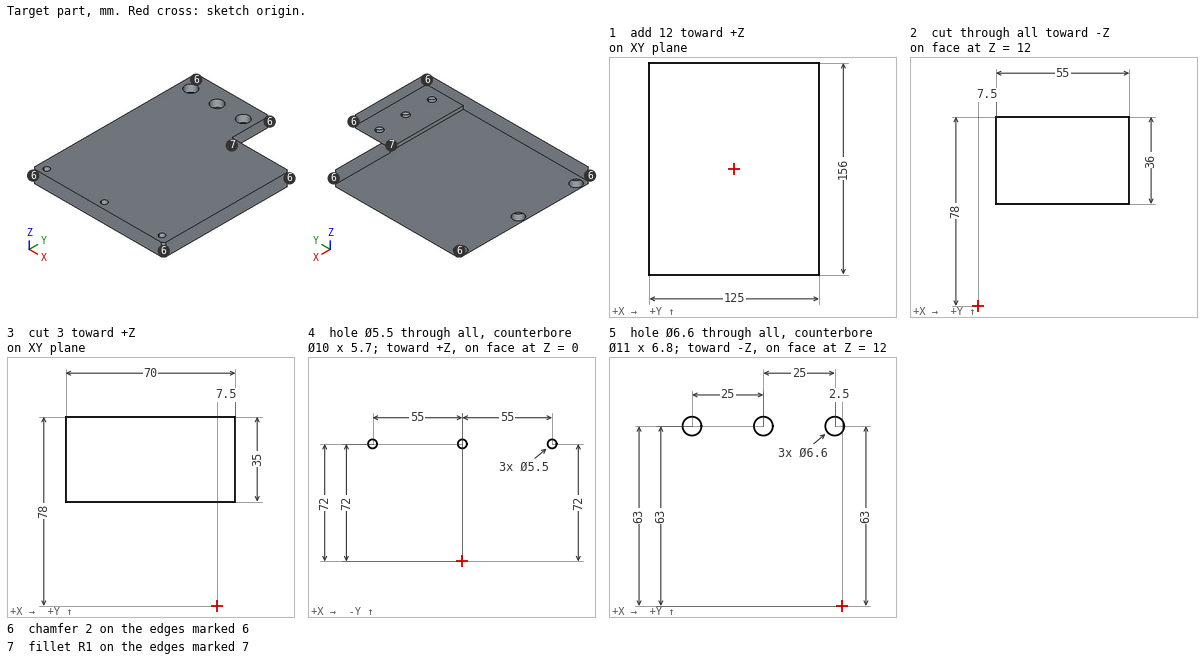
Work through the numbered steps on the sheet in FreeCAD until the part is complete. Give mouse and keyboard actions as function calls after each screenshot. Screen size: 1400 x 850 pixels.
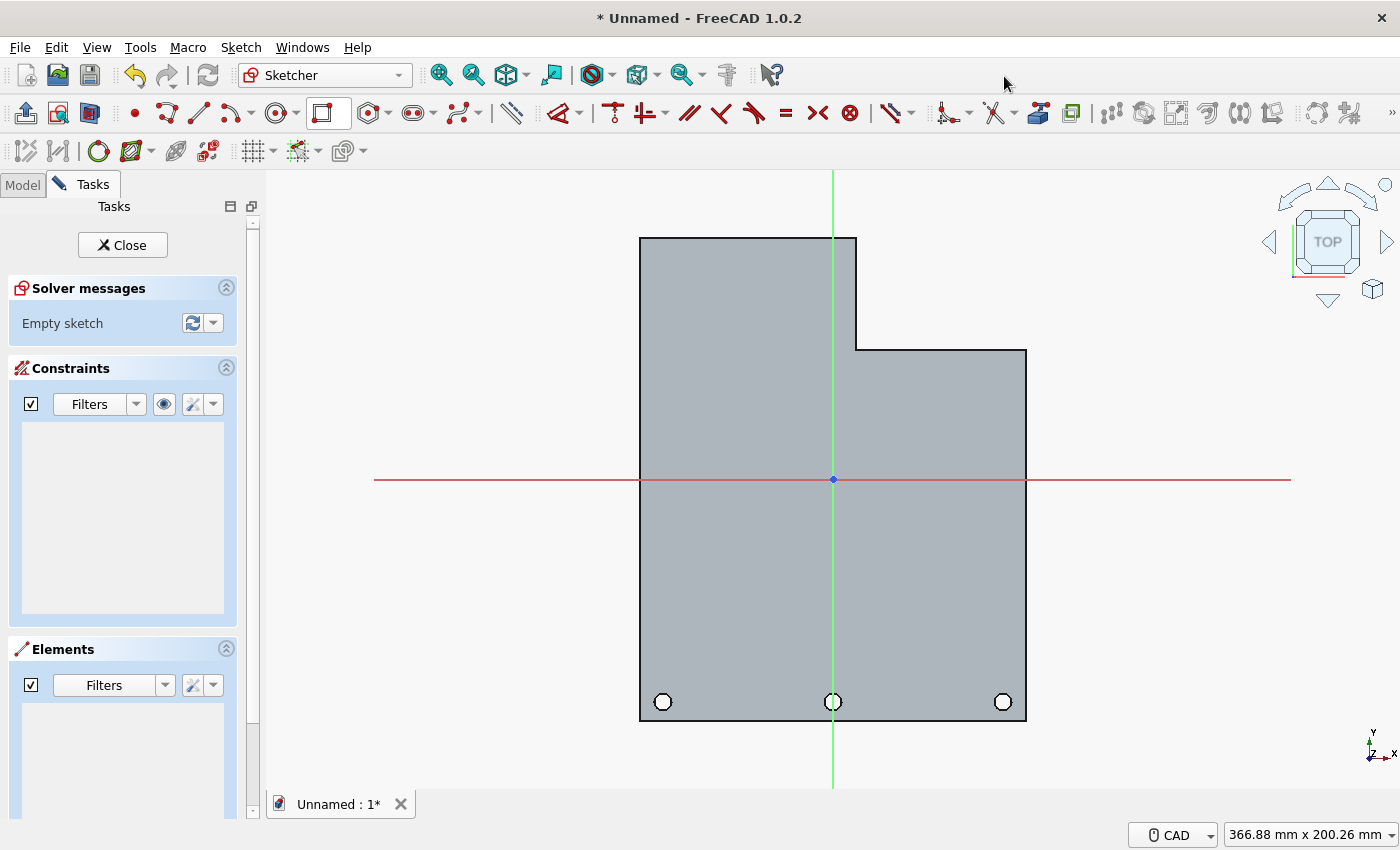
scroll(728, 252, up, 3)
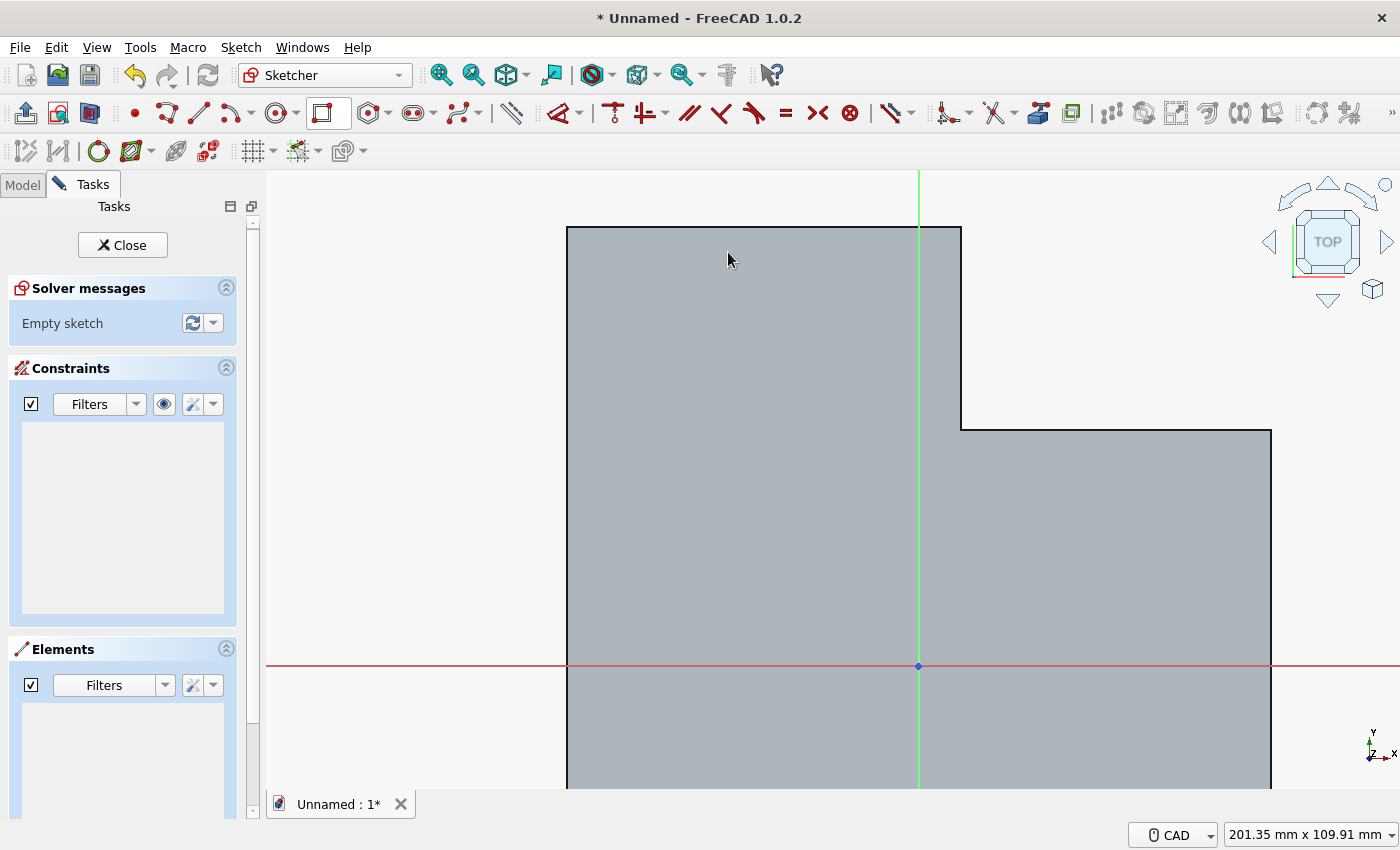
click(276, 114)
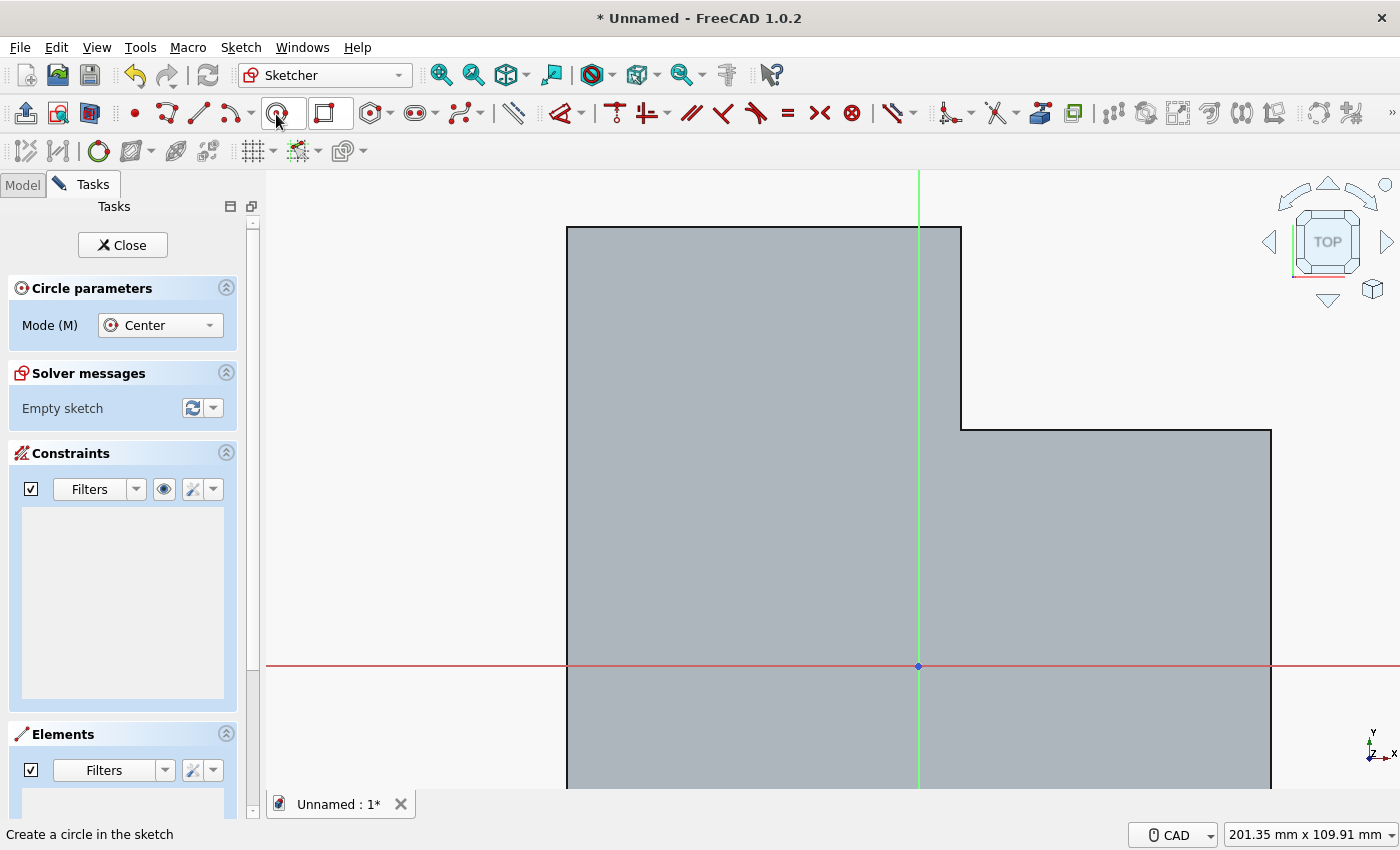
click(905, 312)
move(892, 298)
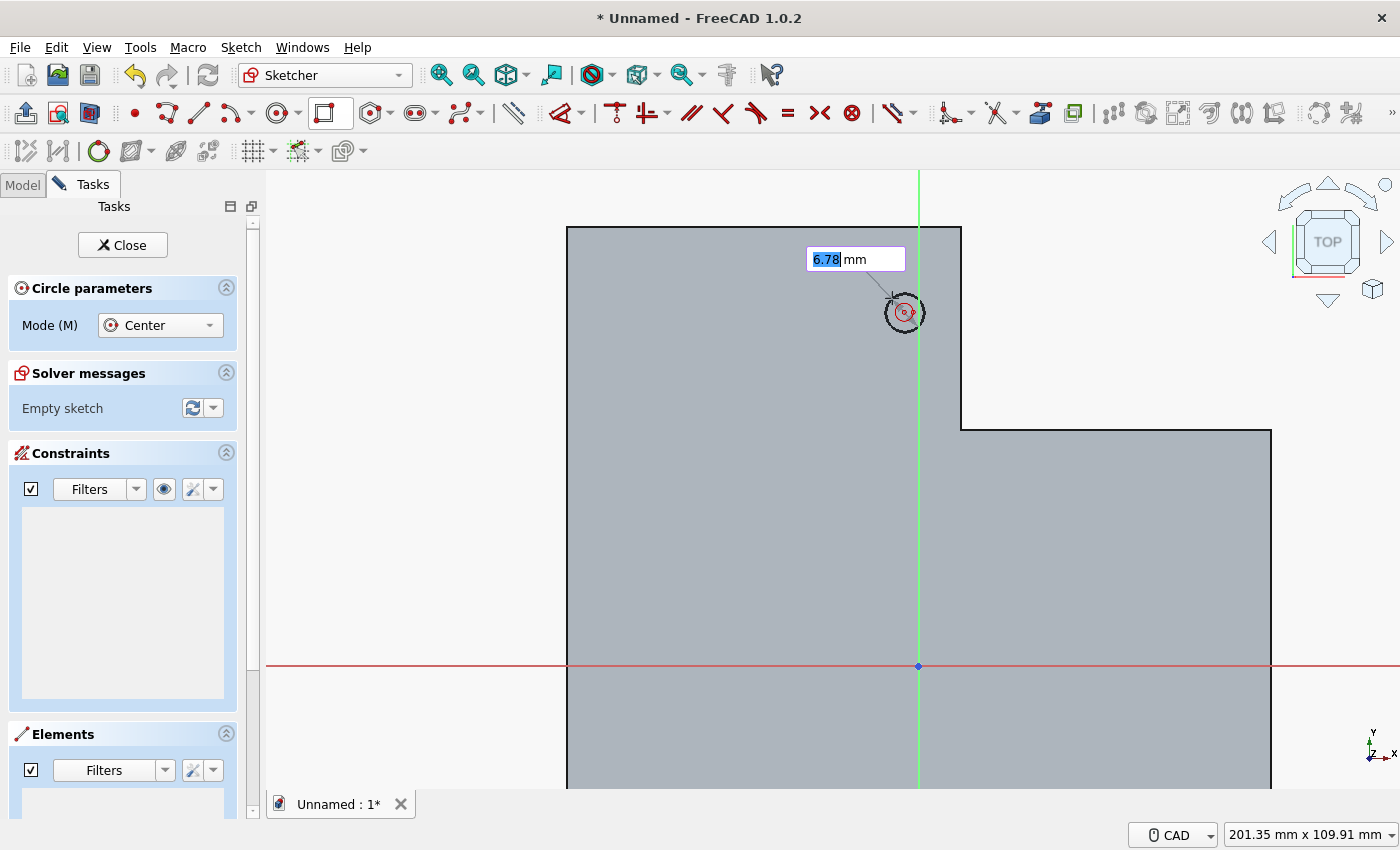
text(6.6)
key(Return)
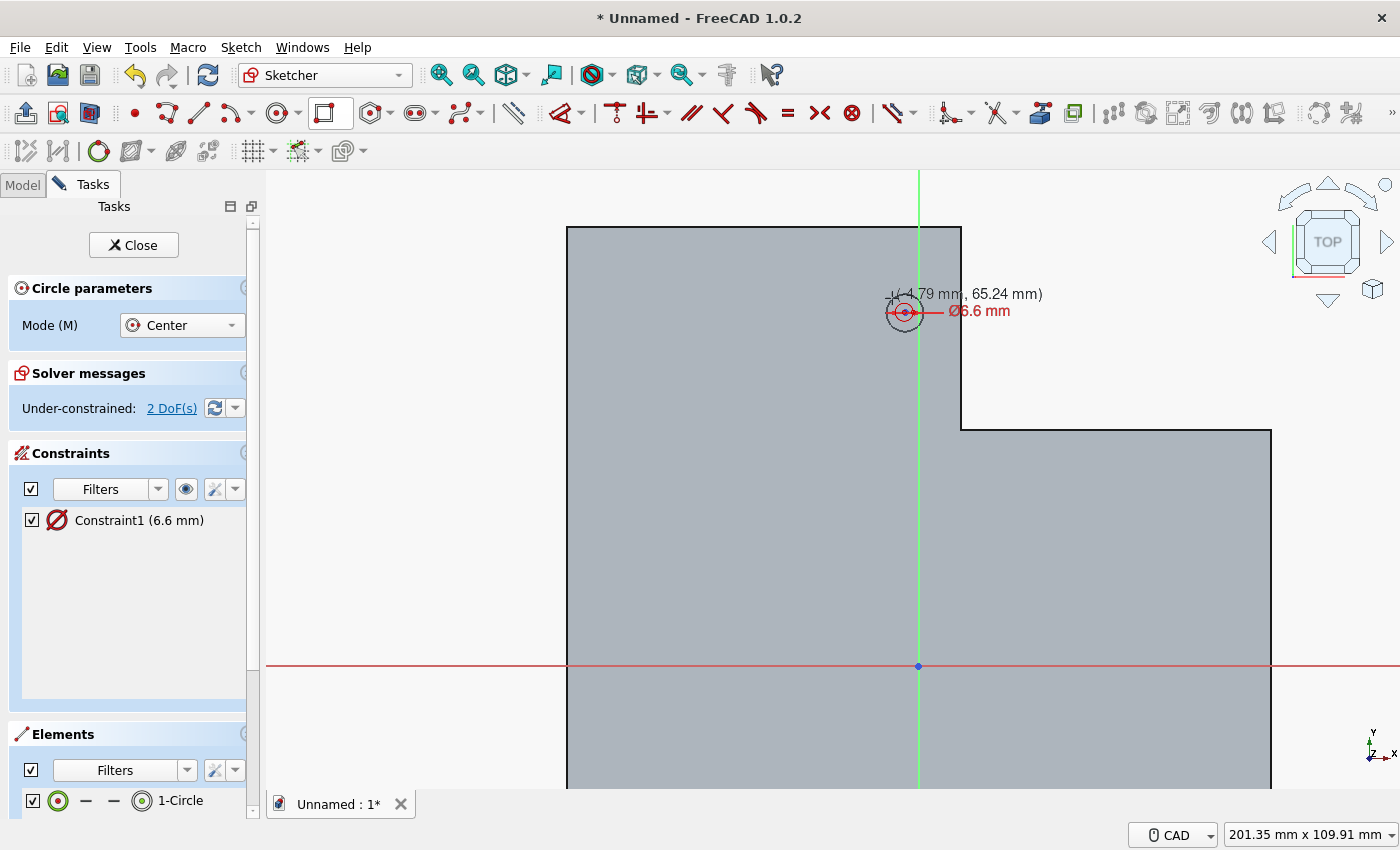
click(764, 312)
move(777, 298)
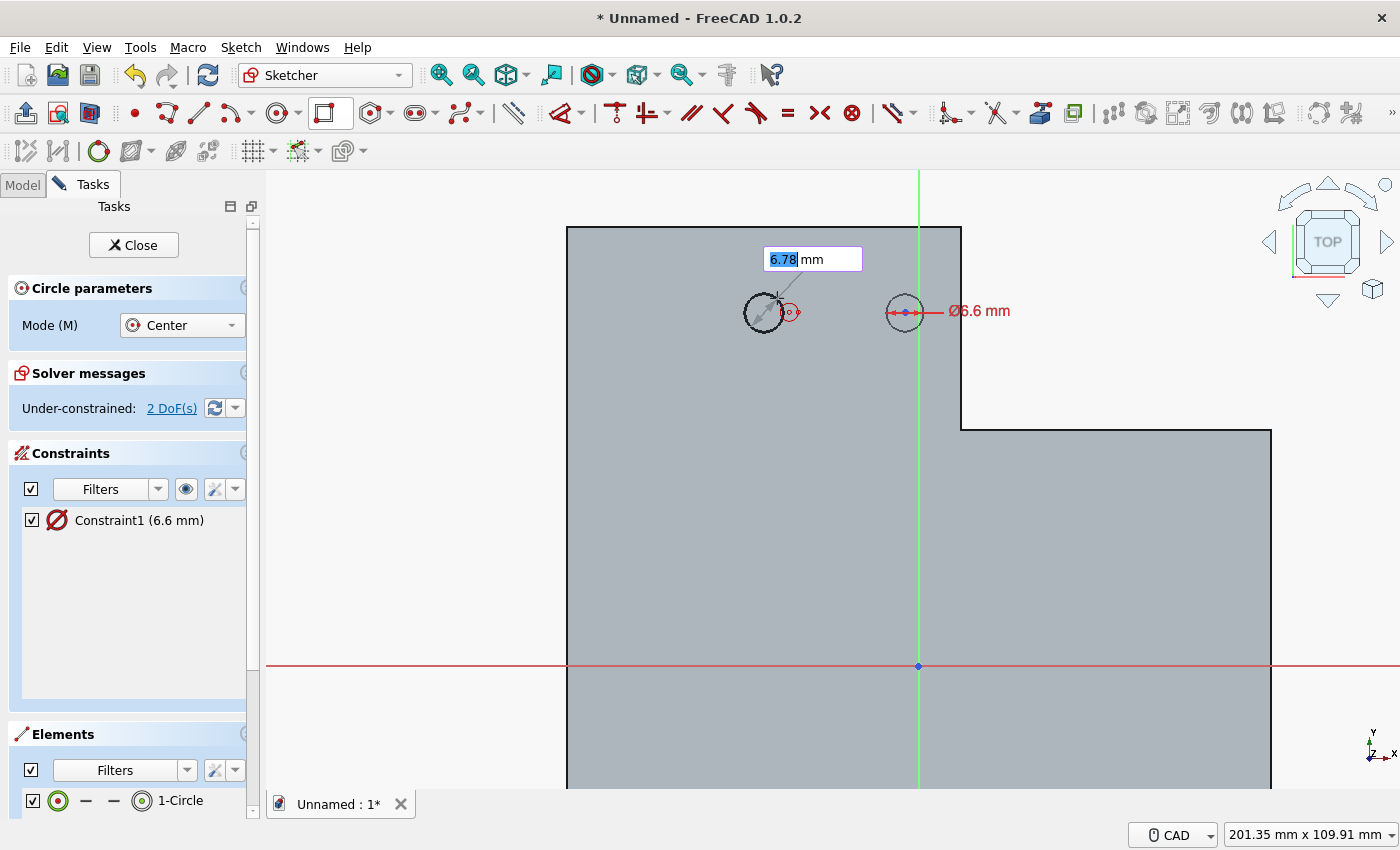
text(6.6)
key(Return)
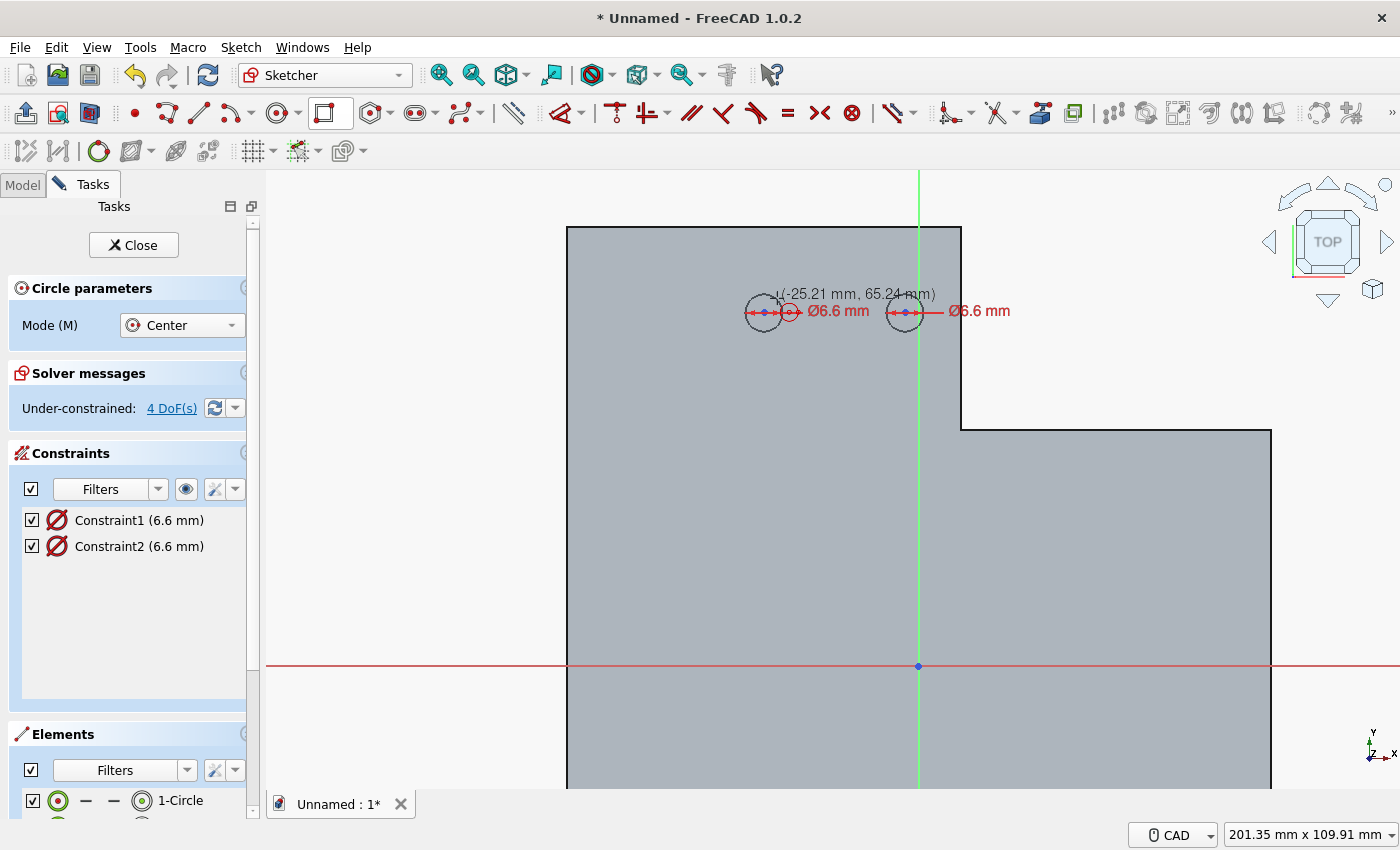
click(623, 312)
move(636, 298)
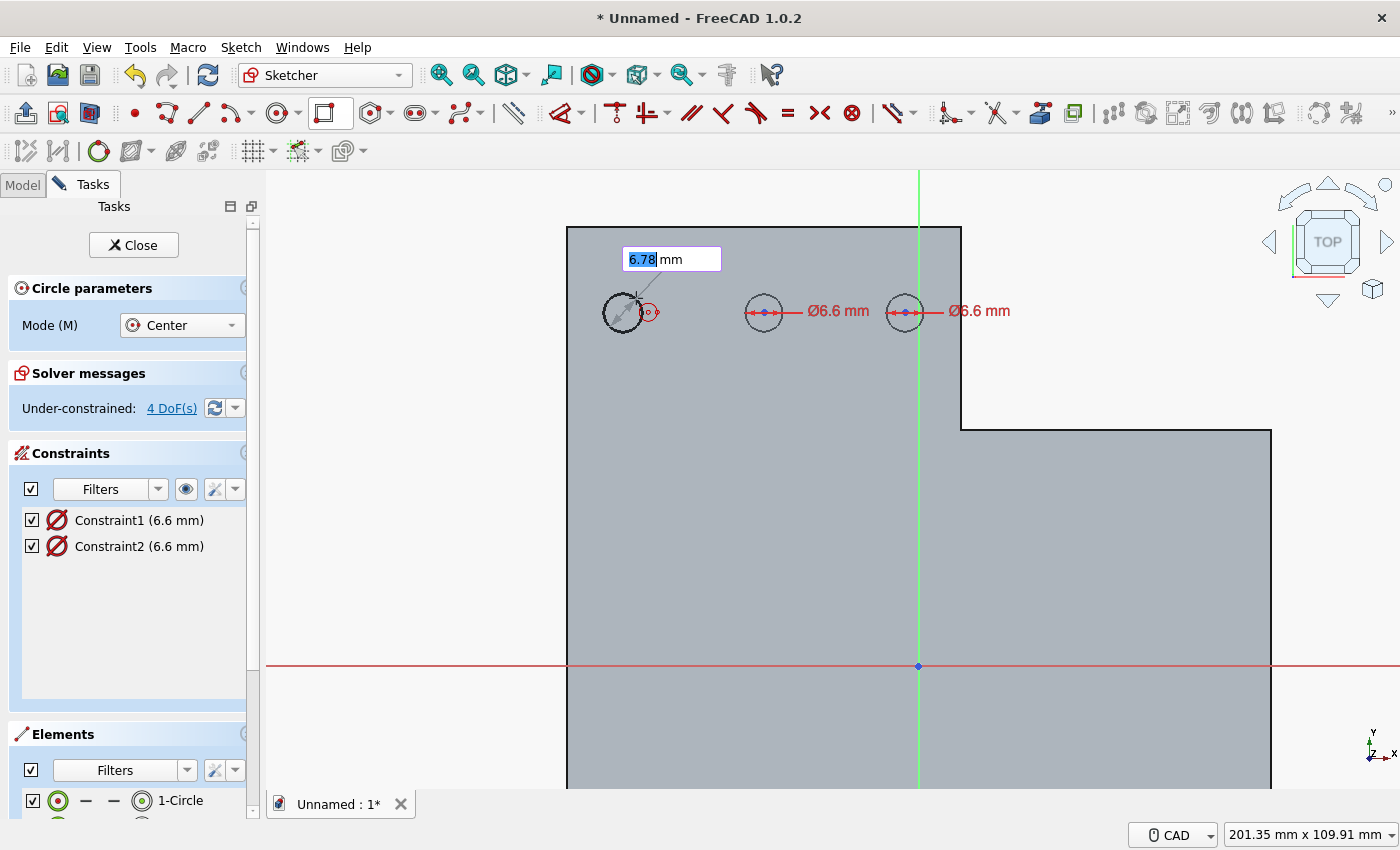
text(6.6)
key(Return)
key(Escape)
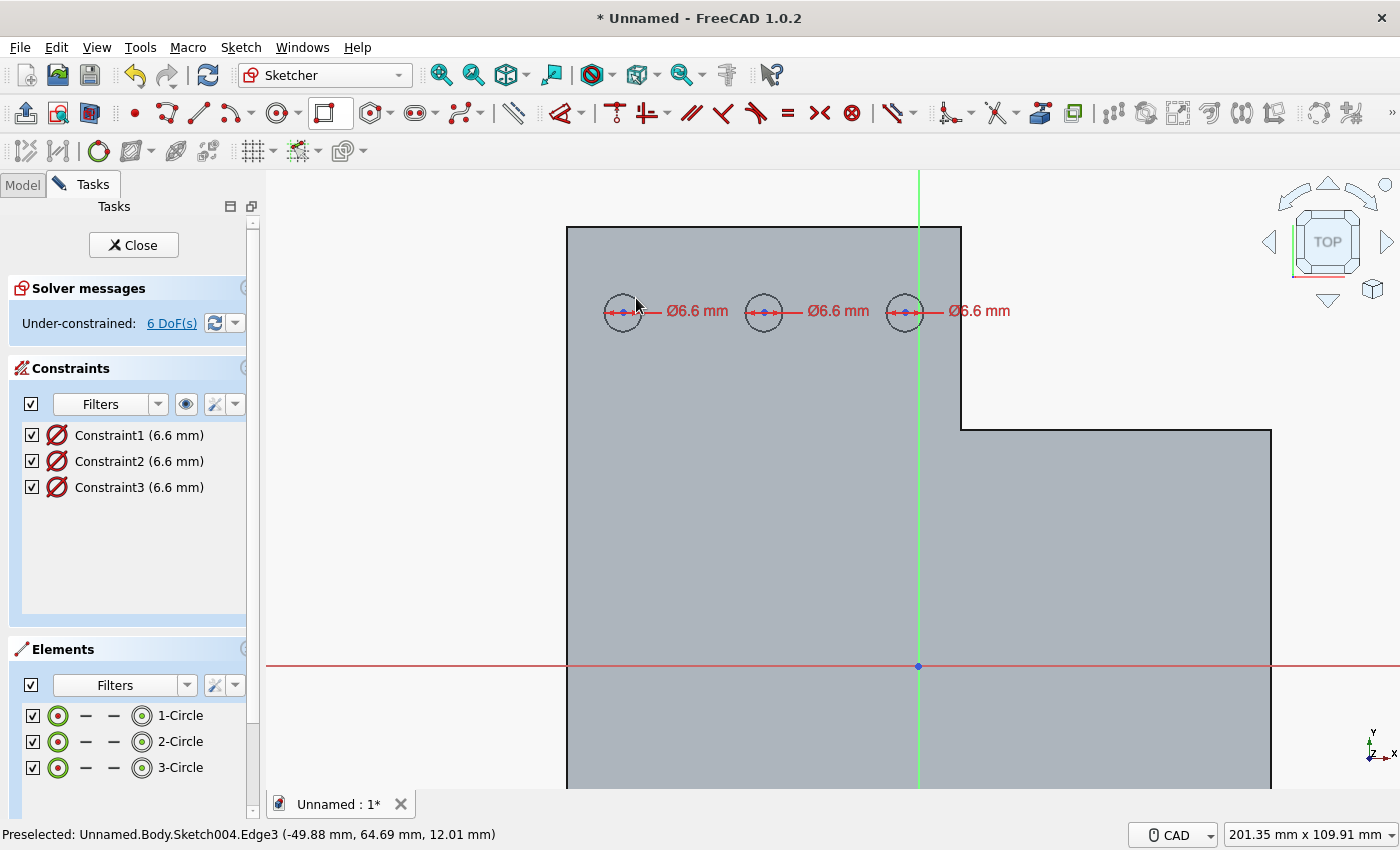
click(560, 114)